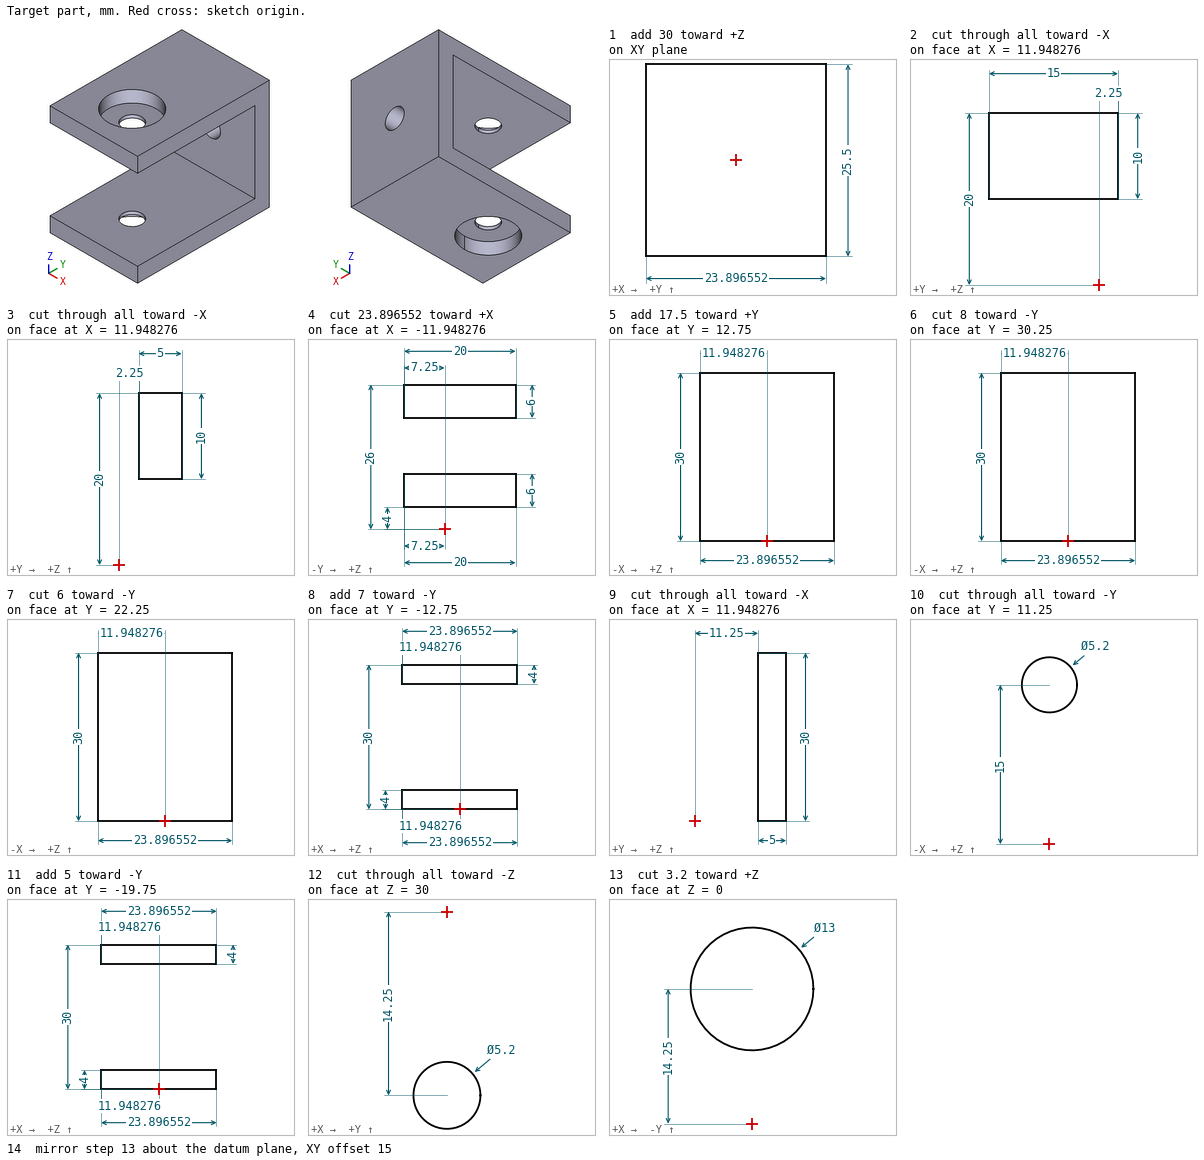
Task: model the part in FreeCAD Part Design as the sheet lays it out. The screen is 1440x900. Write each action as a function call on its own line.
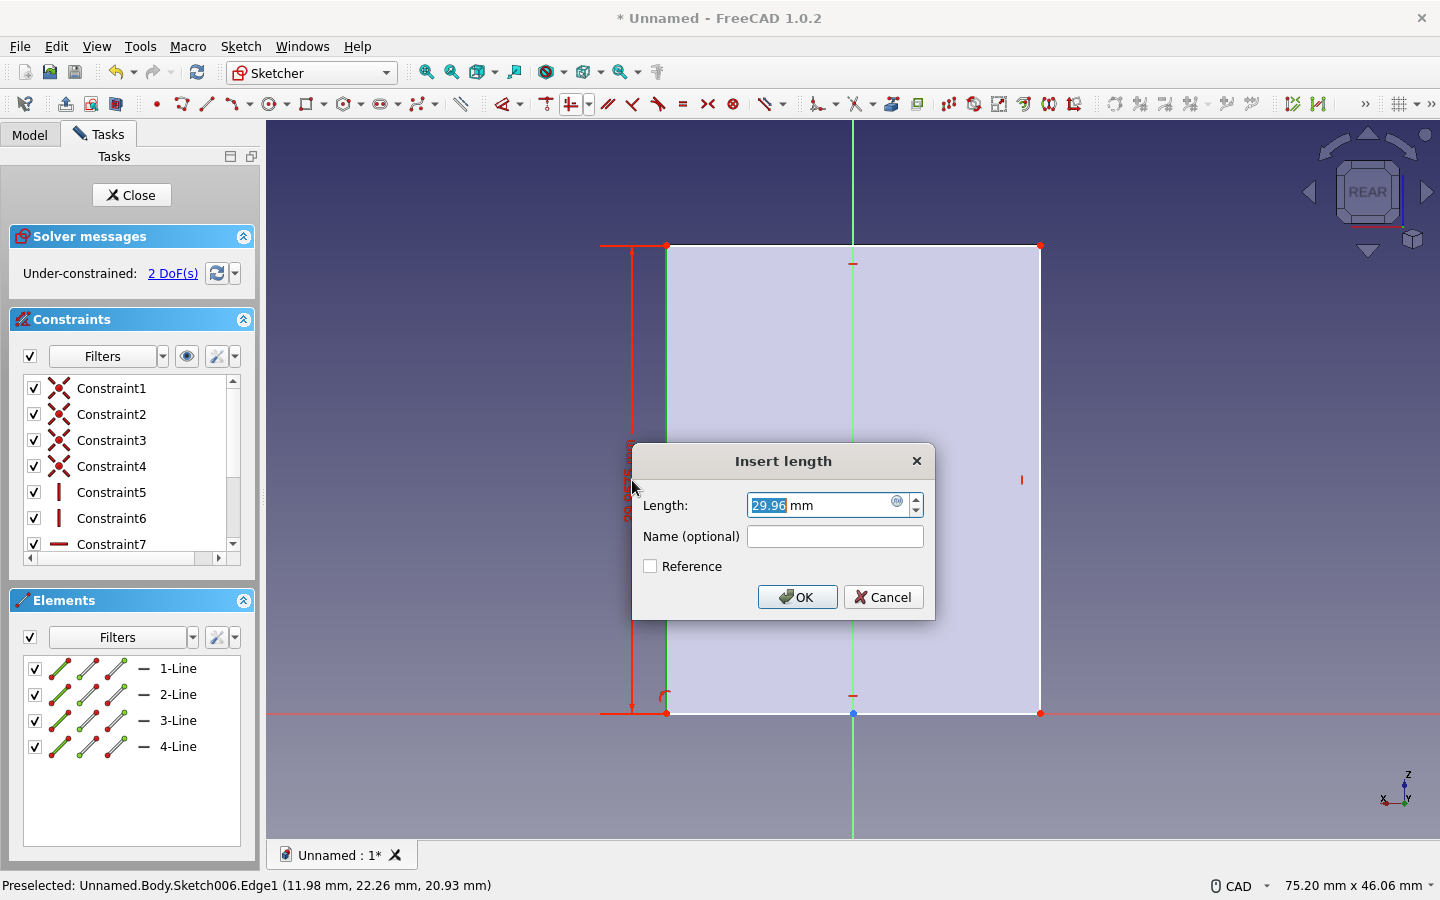
text(30)
key(Return)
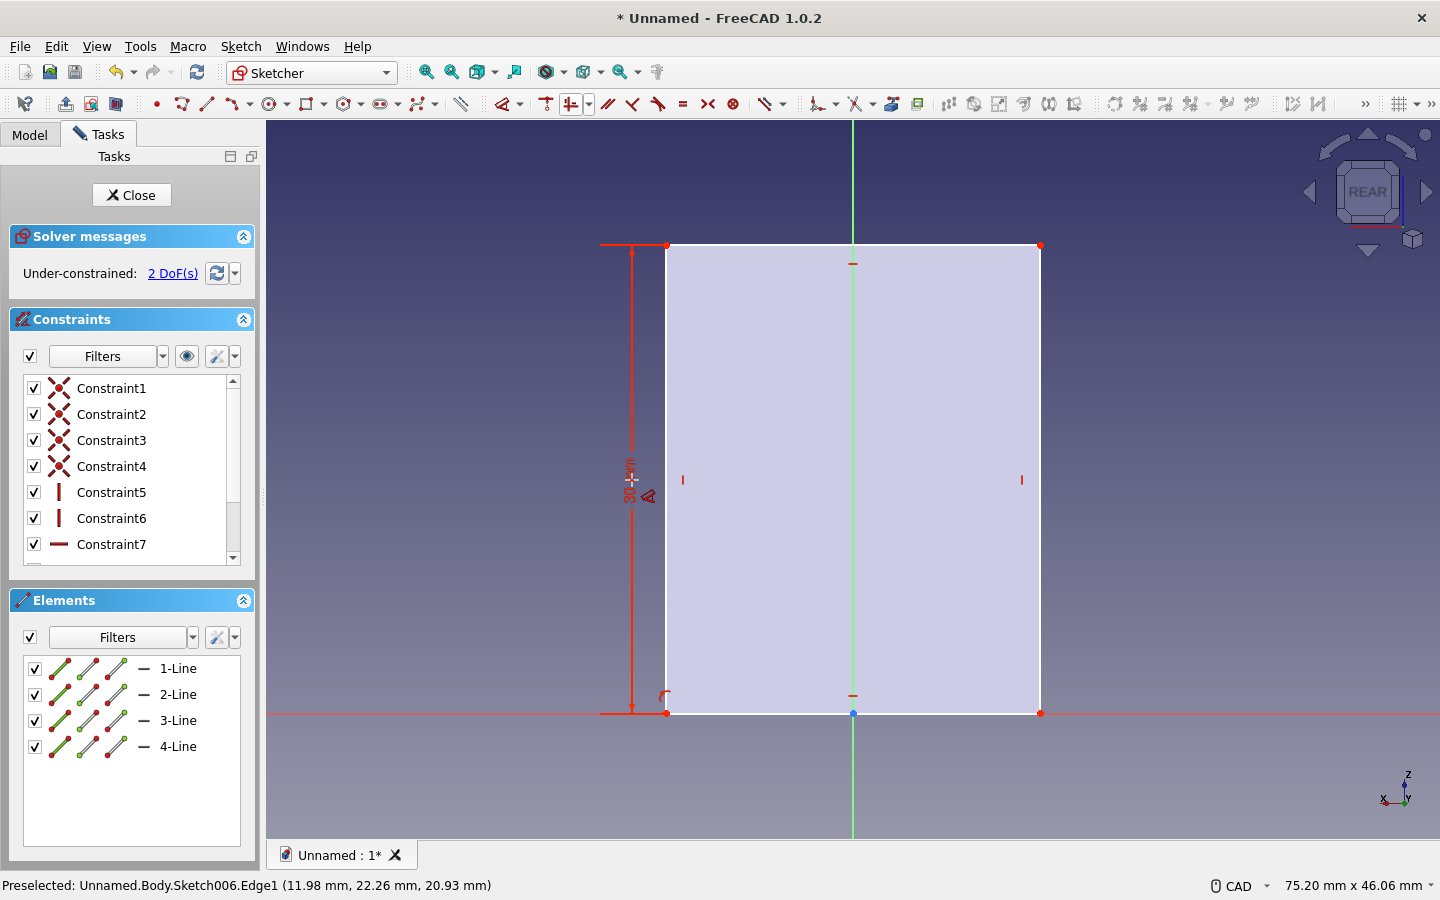
click(778, 714)
click(767, 748)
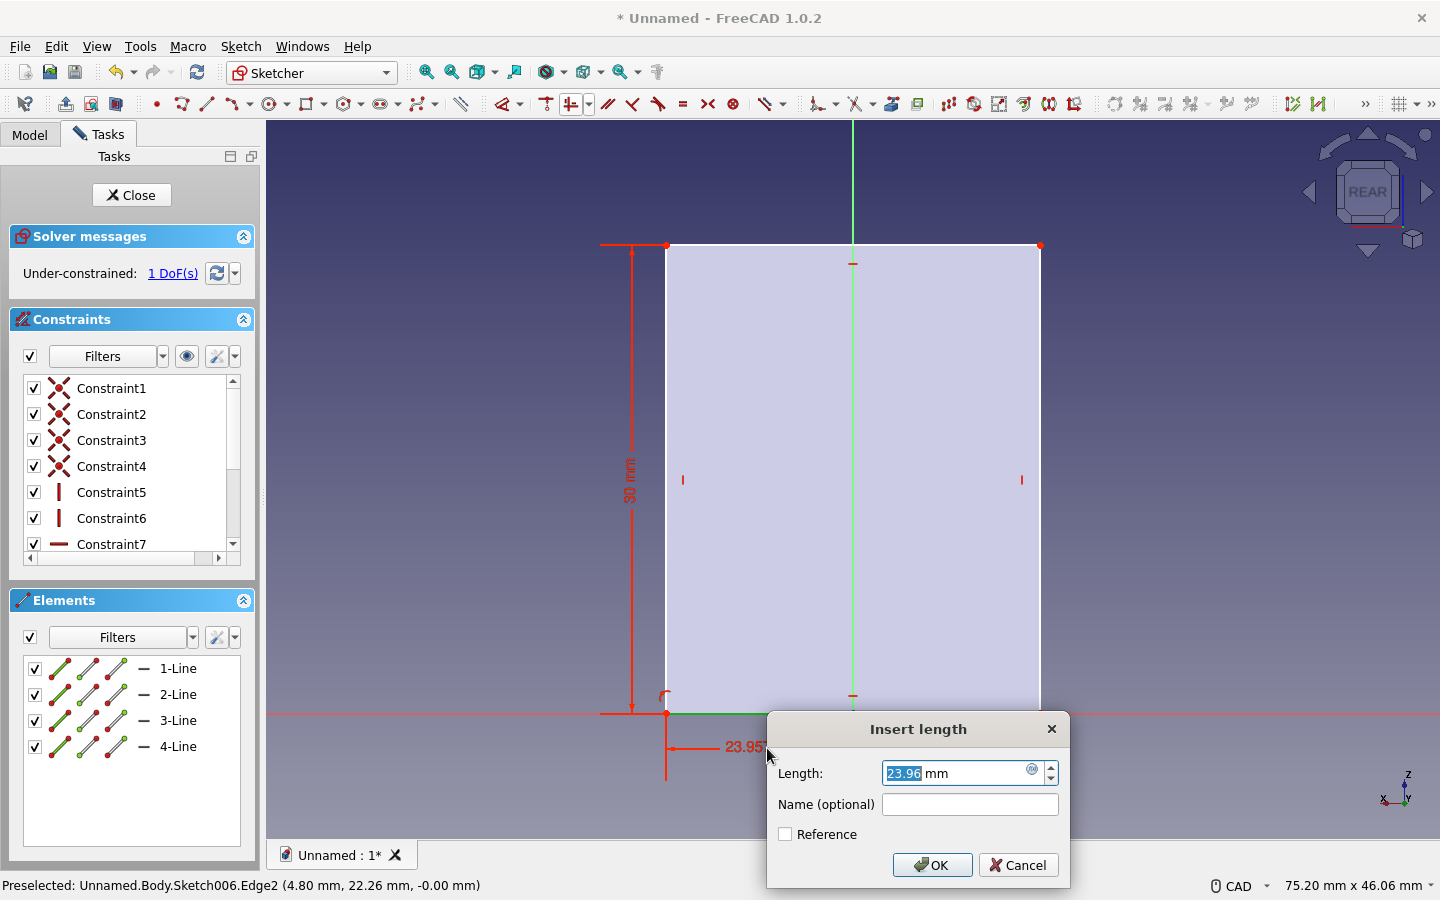
text(23.896552)
key(Return)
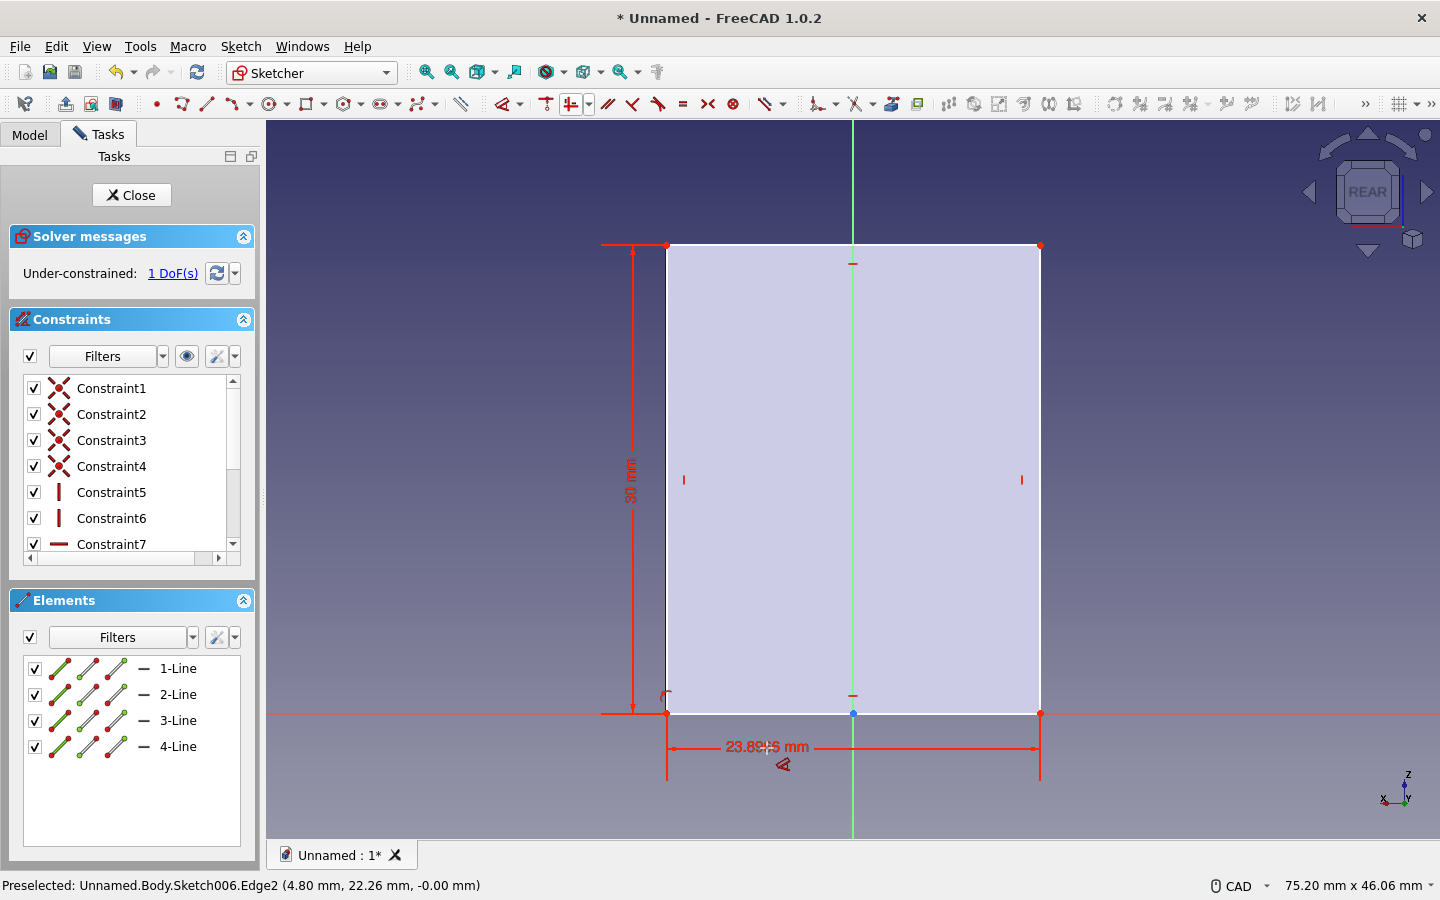
click(667, 245)
click(695, 748)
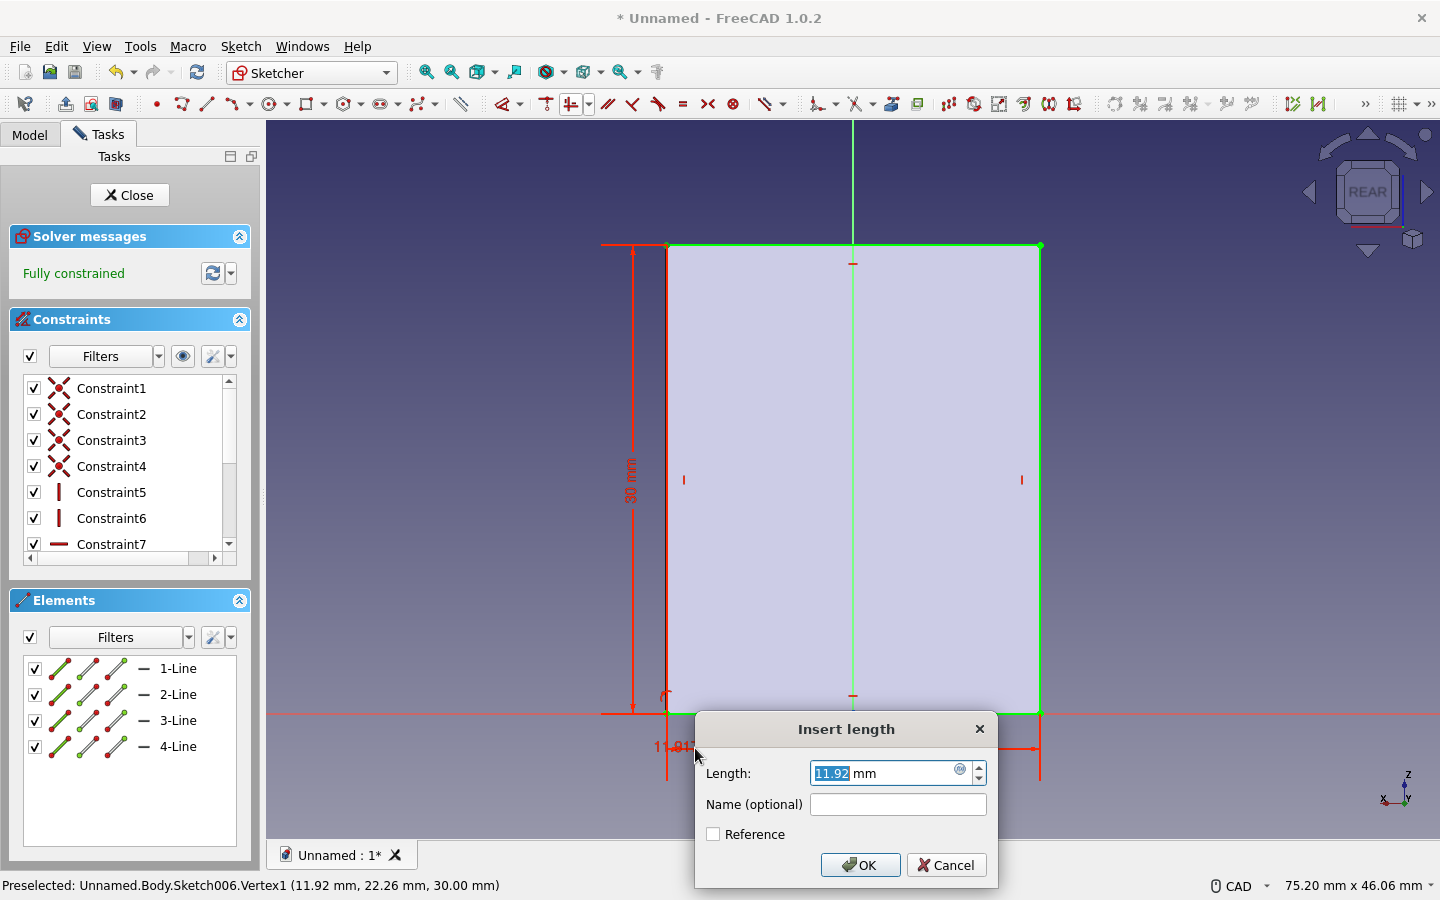
text(11.948276)
key(Return)
key(Escape)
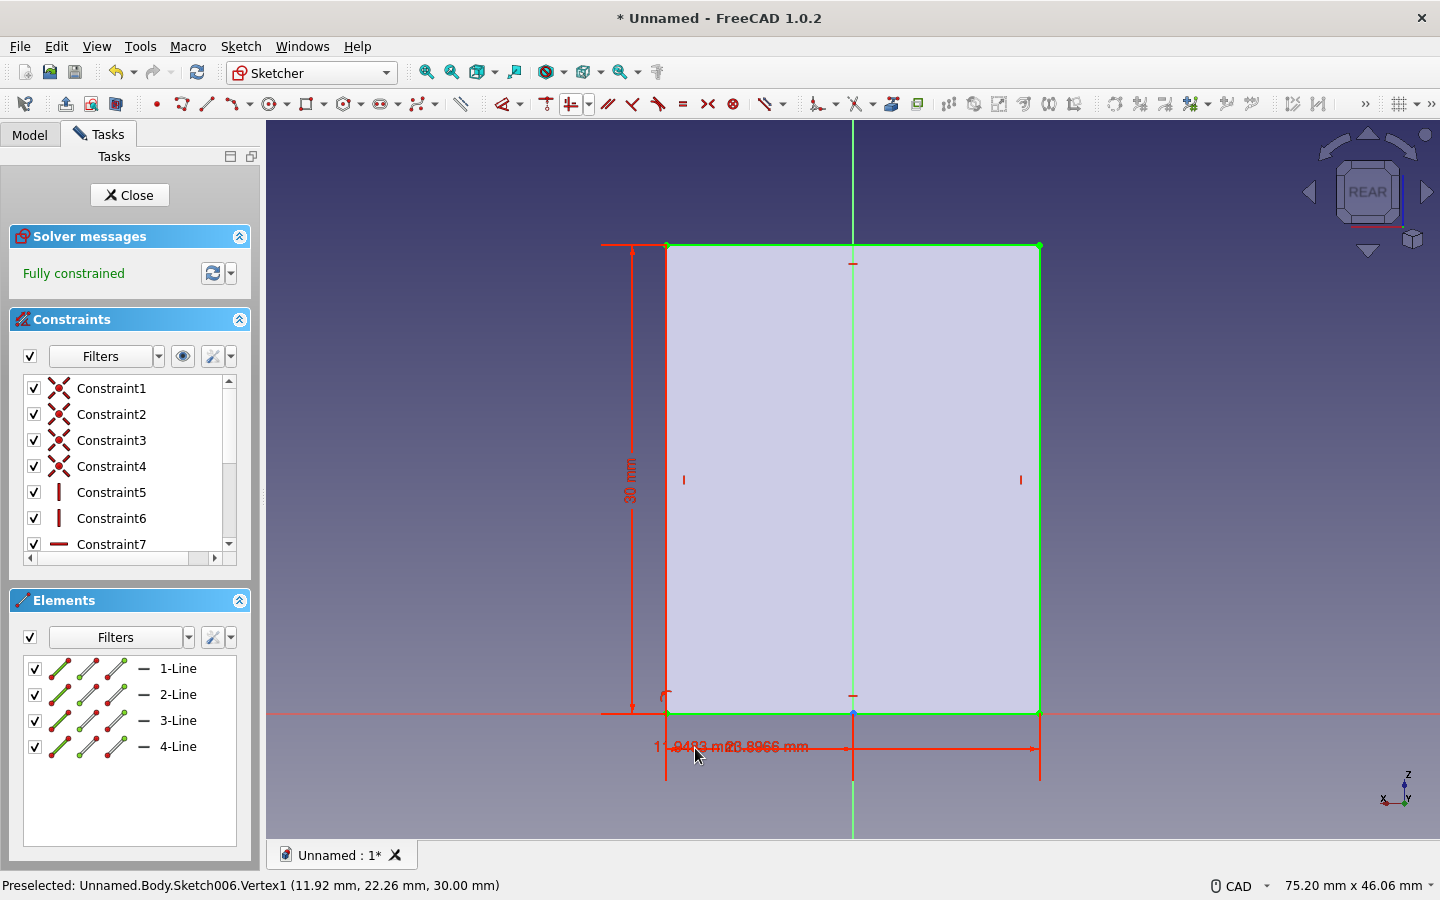
click(130, 195)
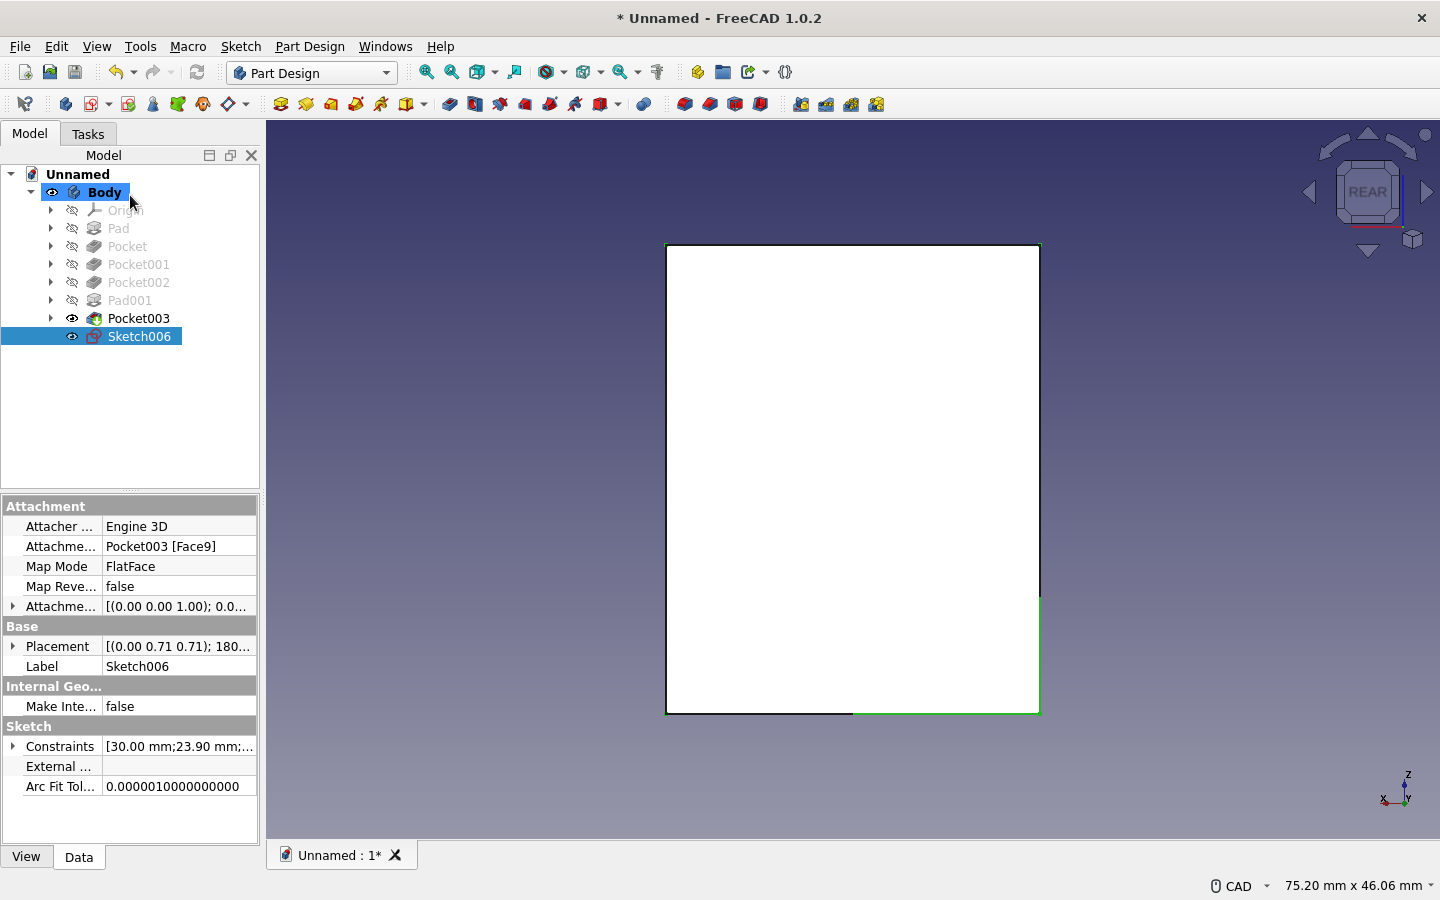
click(450, 104)